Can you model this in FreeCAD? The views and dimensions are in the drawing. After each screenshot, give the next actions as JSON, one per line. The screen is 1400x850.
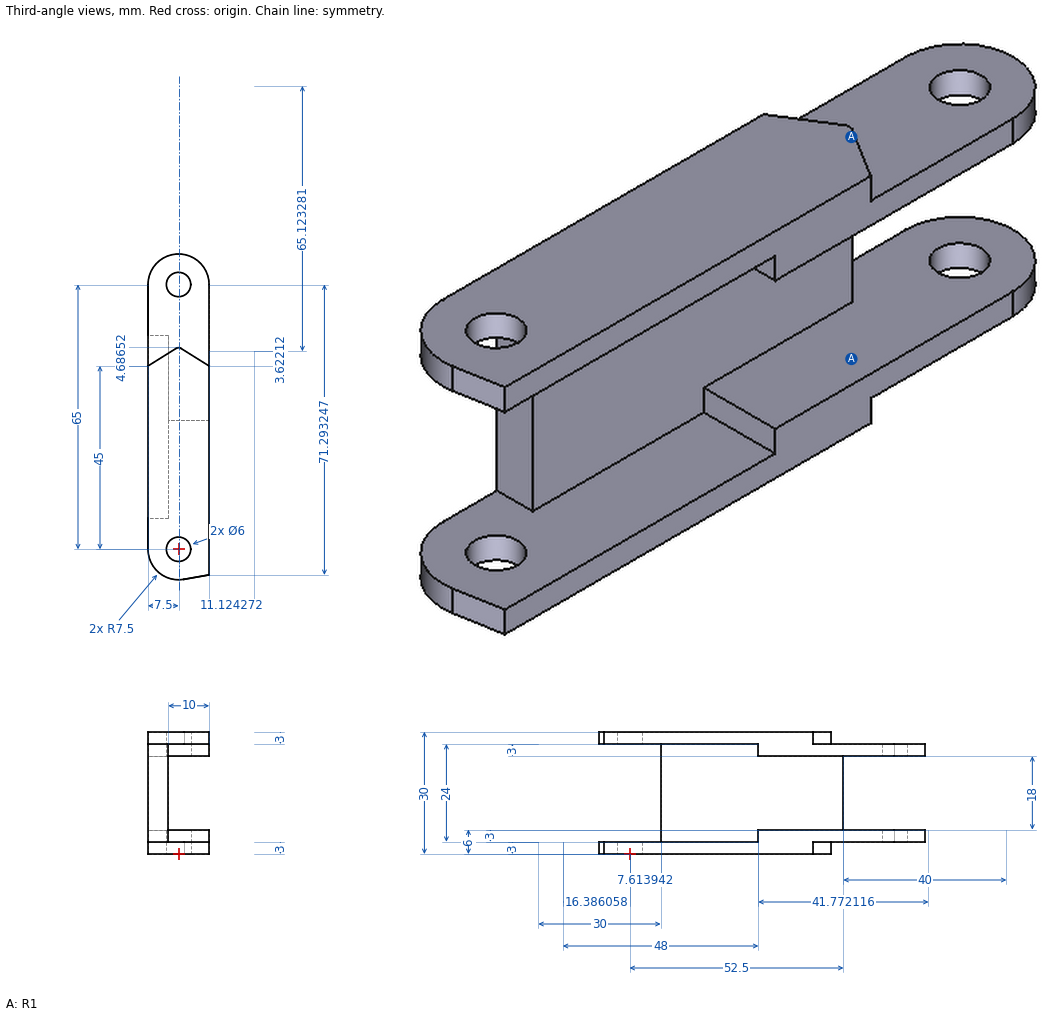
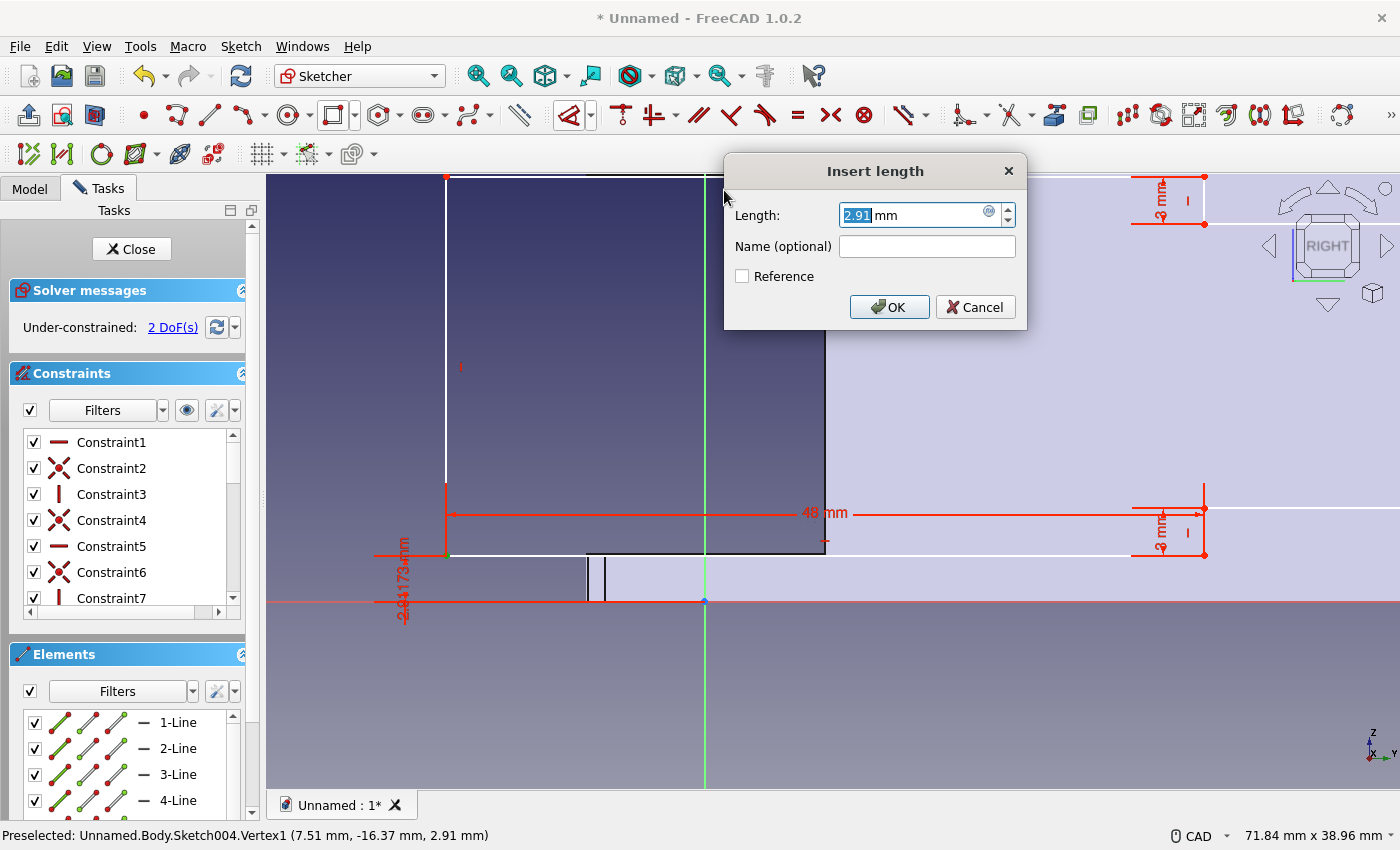
{"action": "type", "text": "3"}
{"action": "key", "text": "Return"}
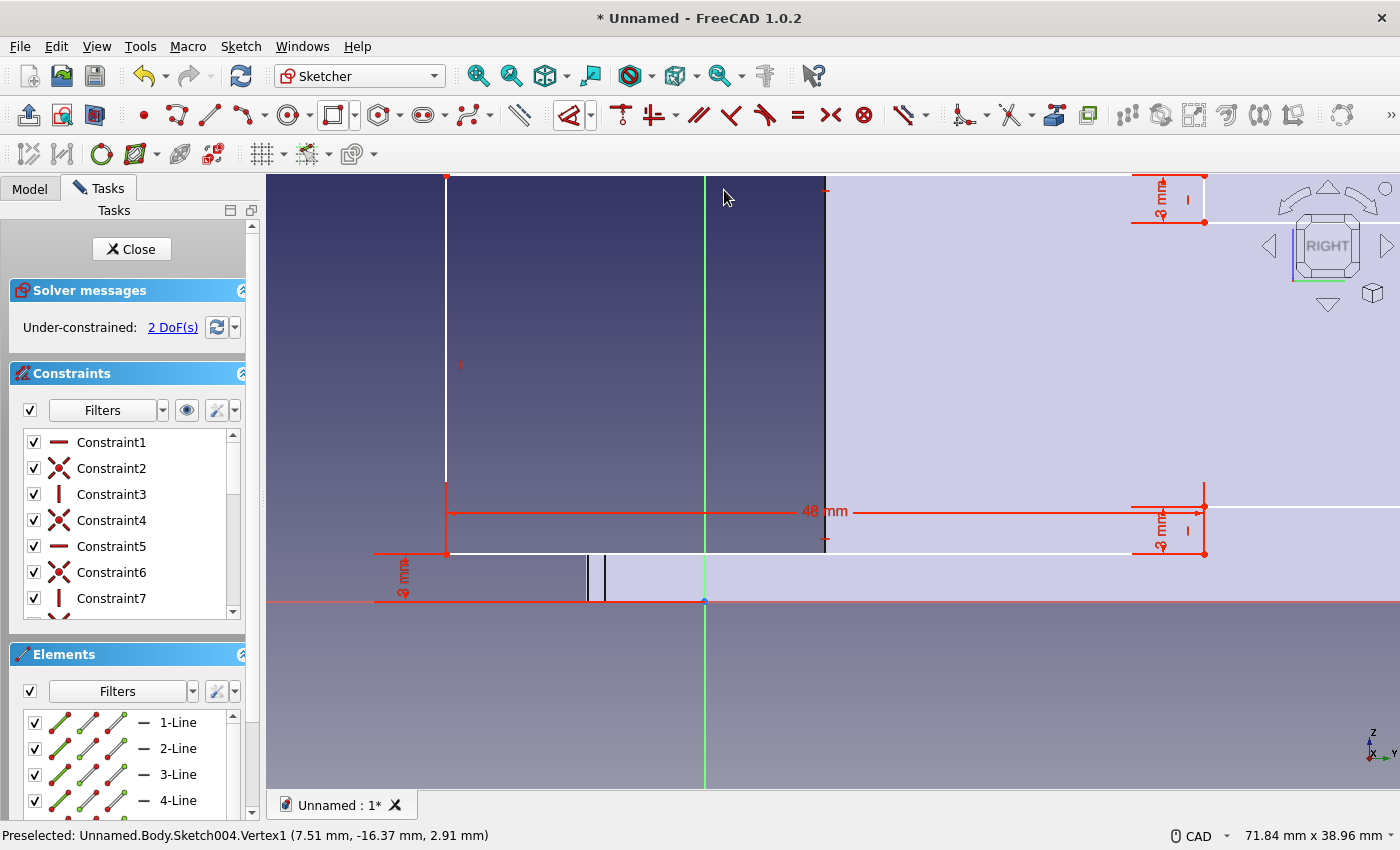
{"action": "scroll", "coordinate": [446, 557], "scroll_direction": "down", "scroll_amount": 4}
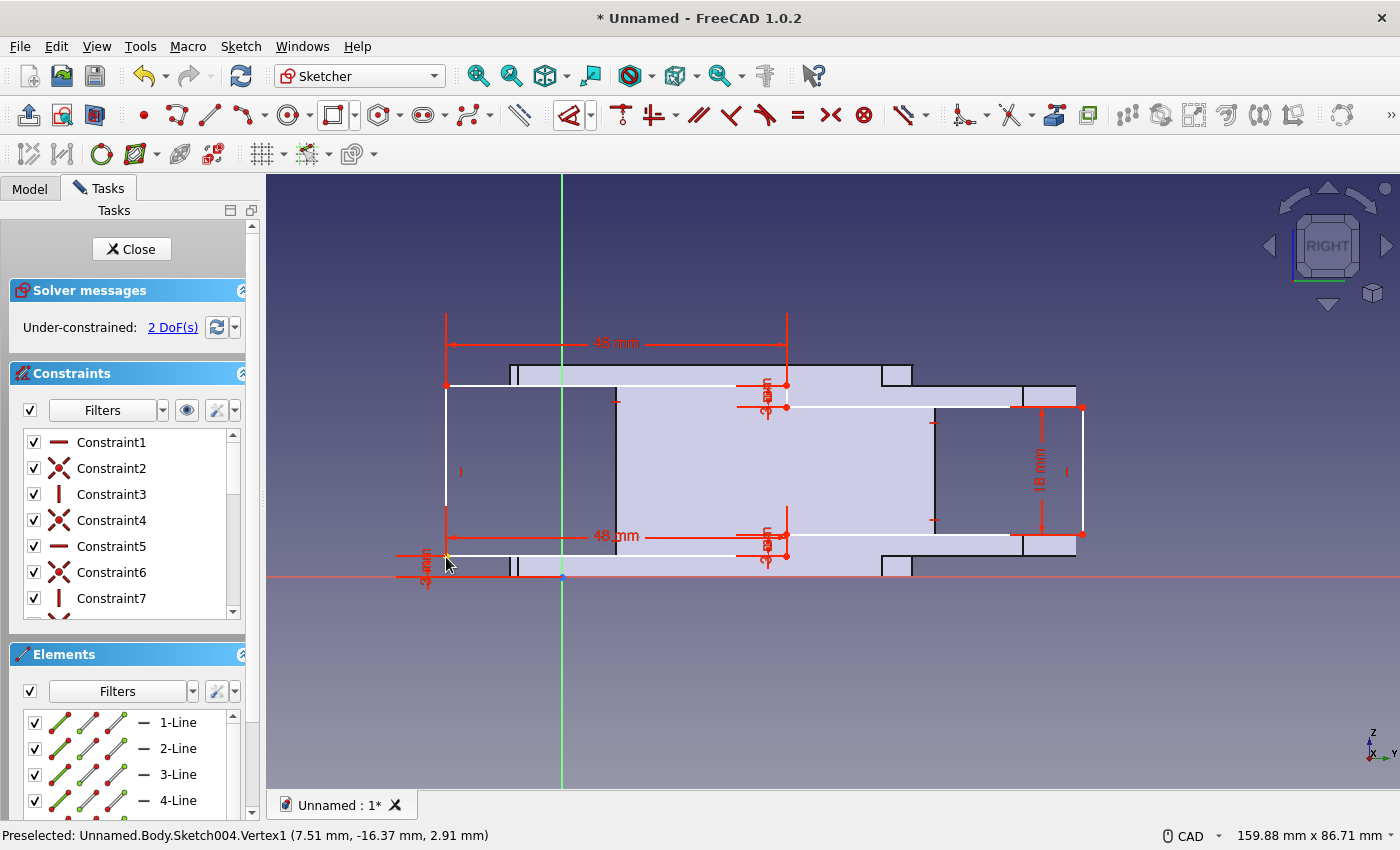
{"action": "left_click", "coordinate": [876, 535]}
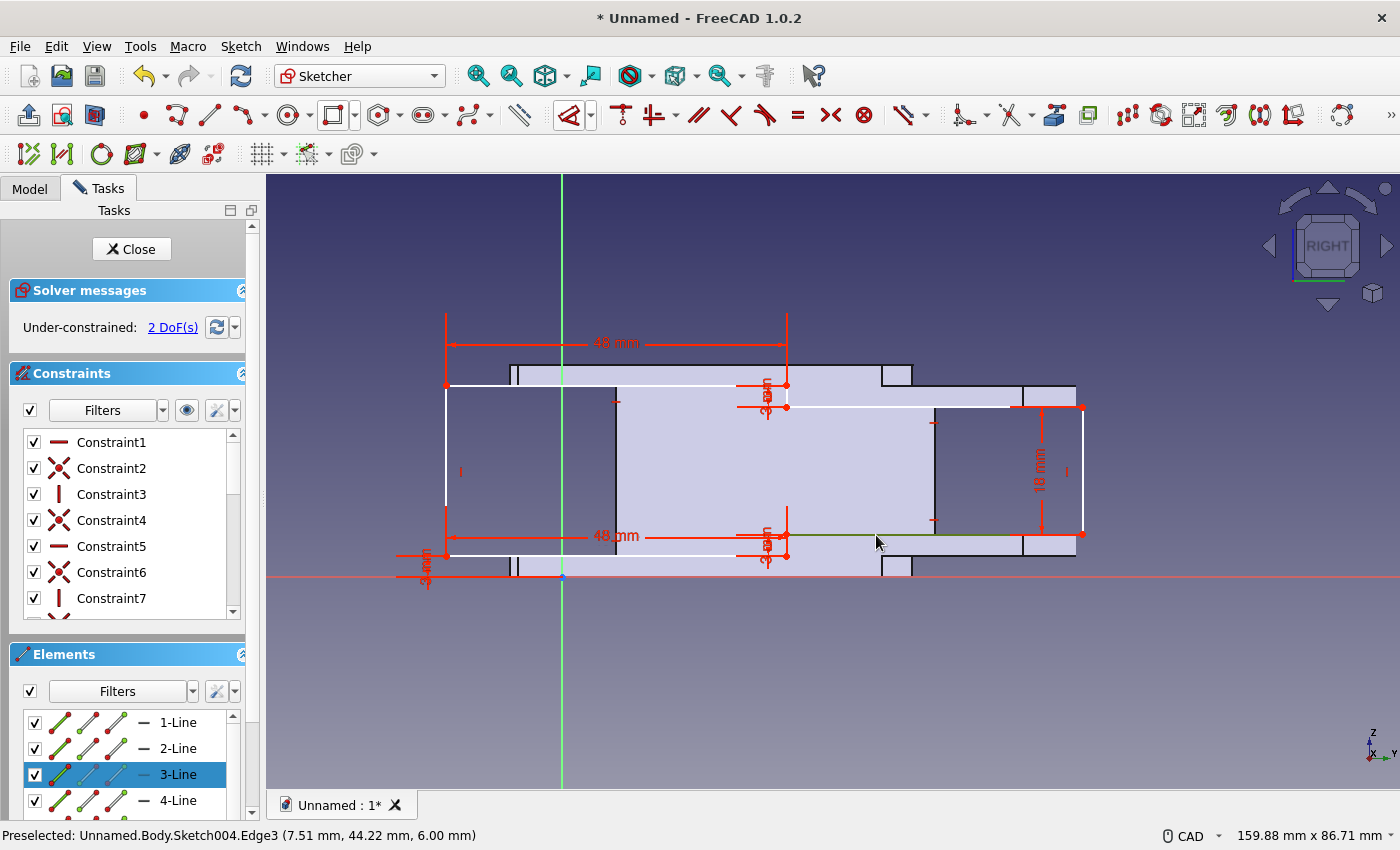
{"action": "left_click", "coordinate": [590, 116]}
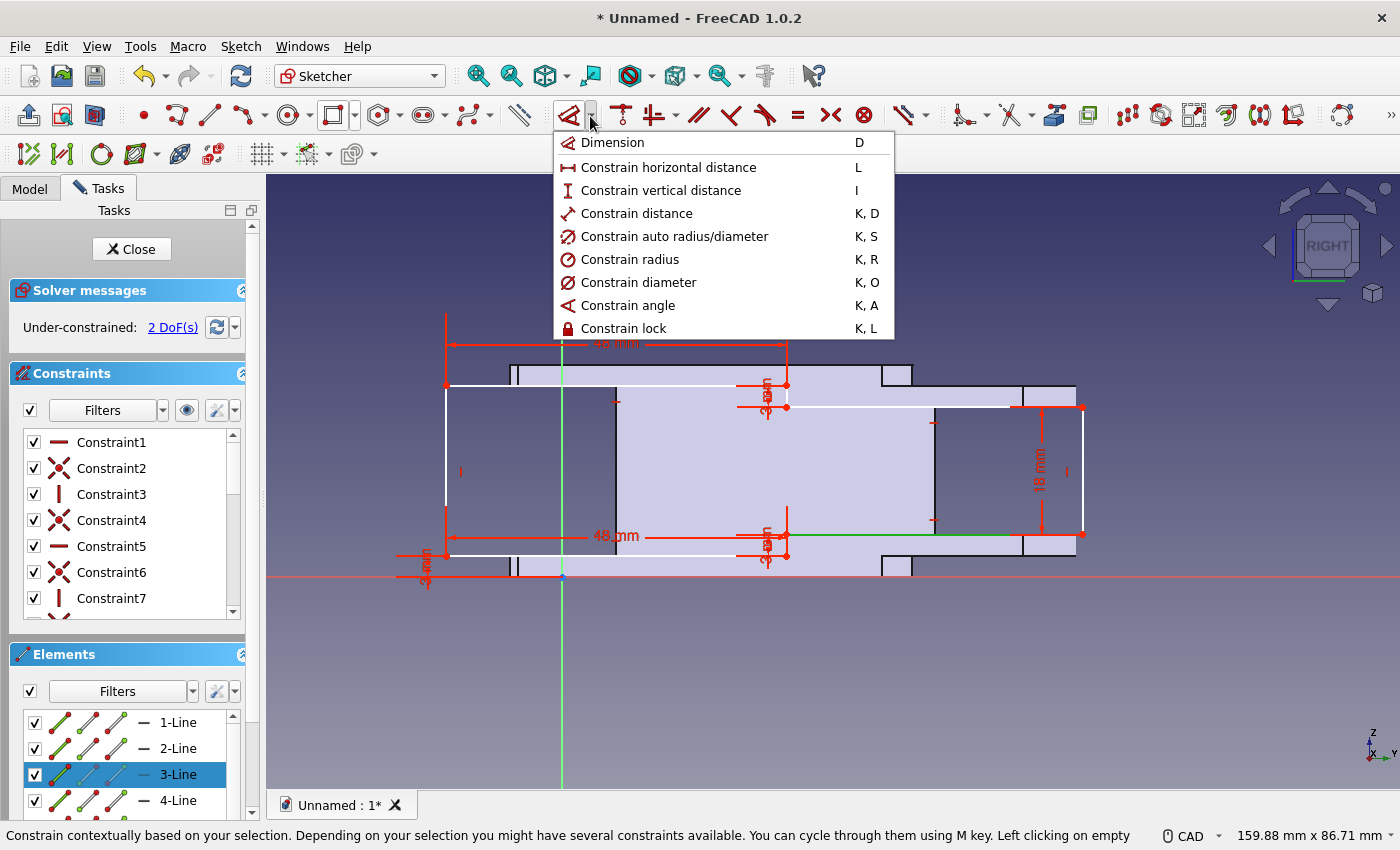
{"action": "left_click", "coordinate": [724, 168]}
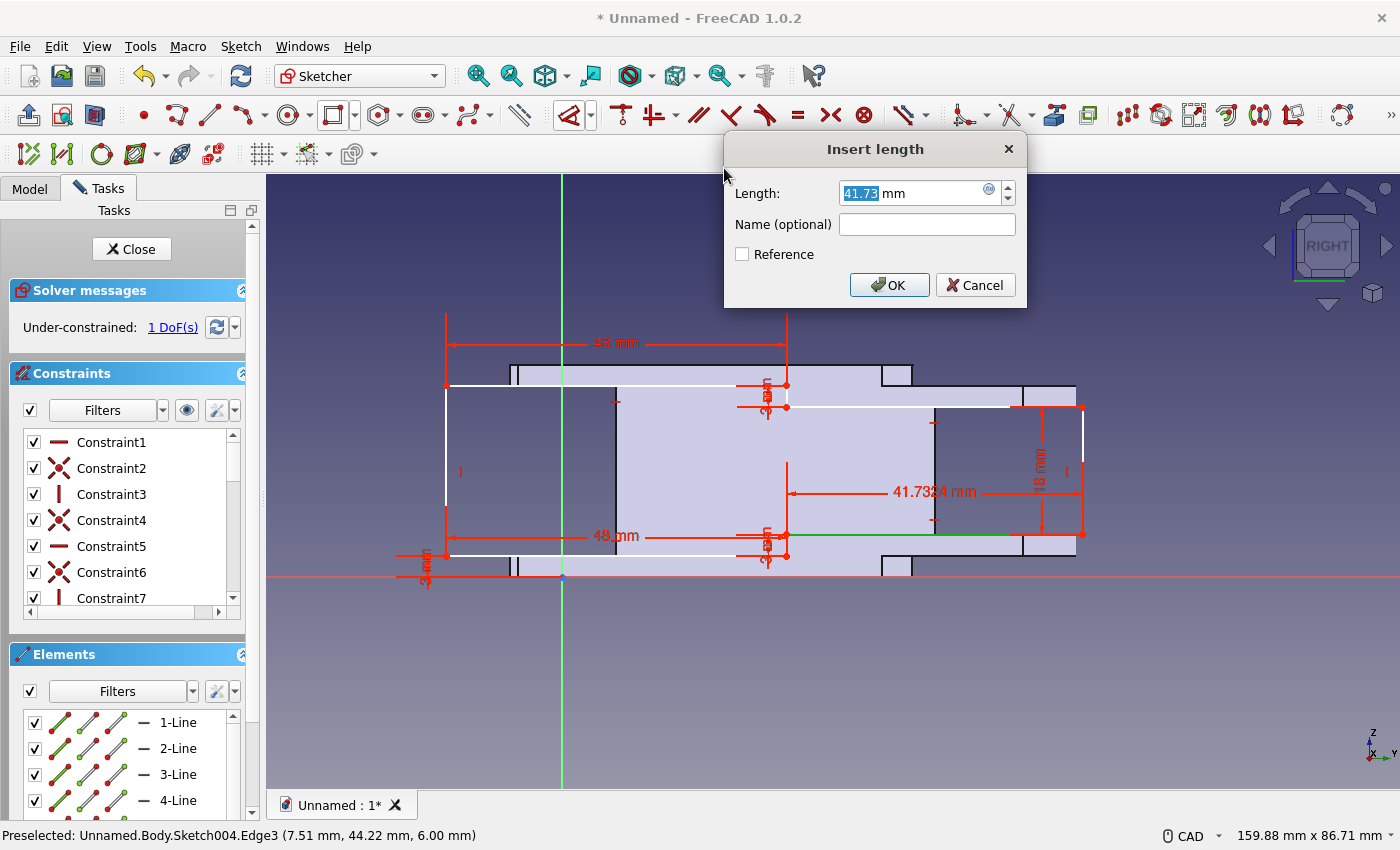
{"action": "type", "text": "41.772116"}
{"action": "key", "text": "Return"}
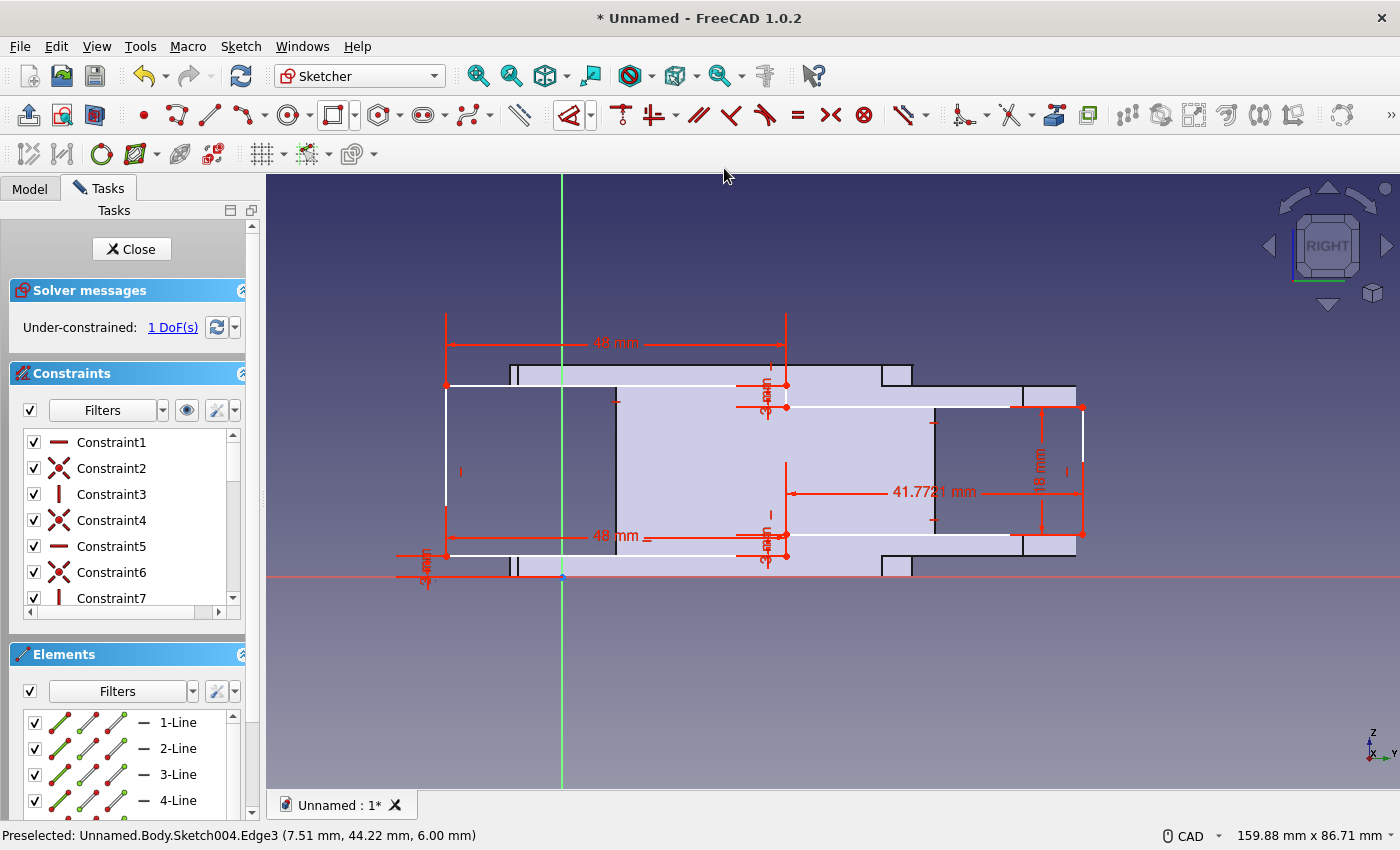
{"action": "left_click", "coordinate": [446, 556]}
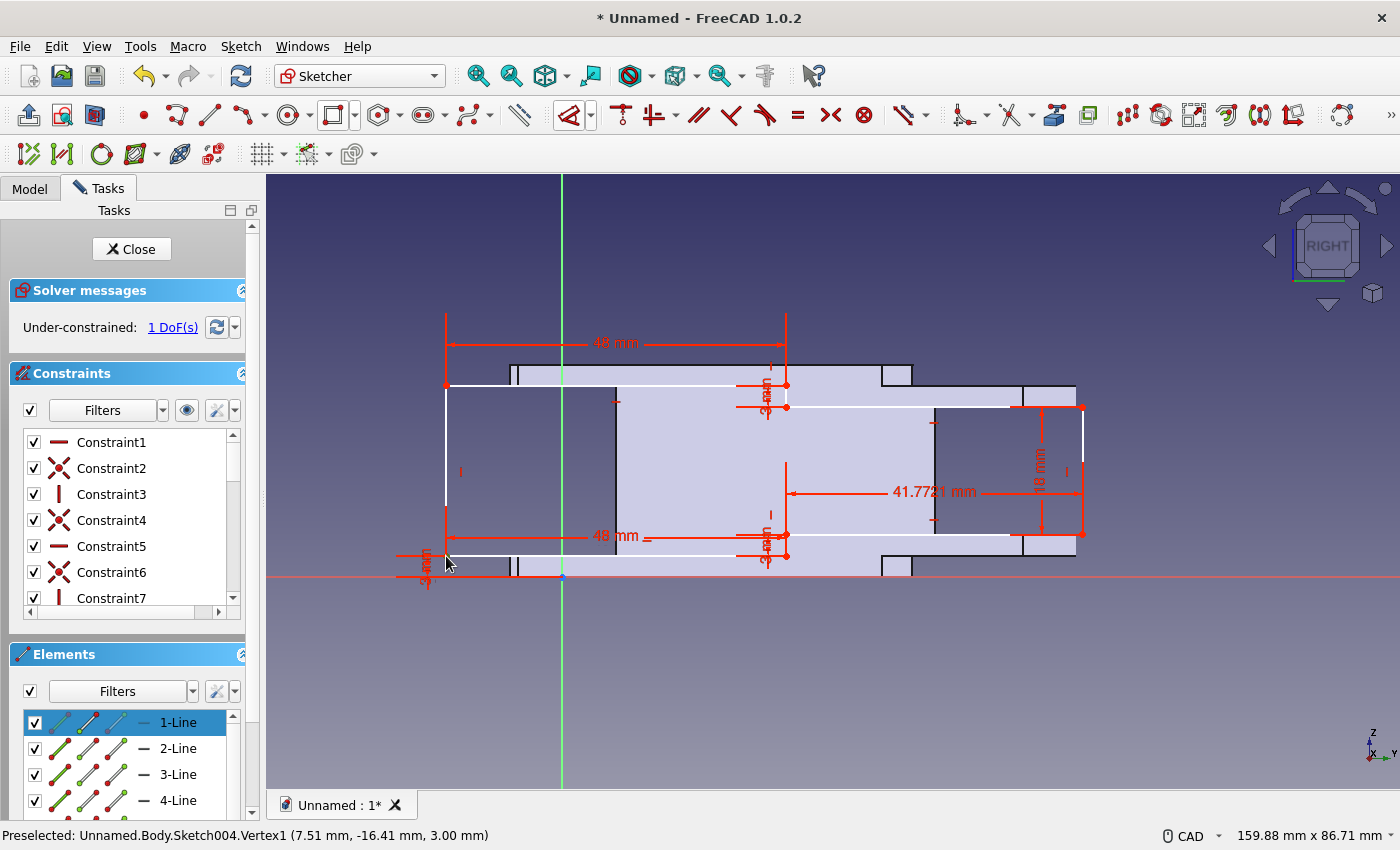
{"action": "key", "text": "l"}